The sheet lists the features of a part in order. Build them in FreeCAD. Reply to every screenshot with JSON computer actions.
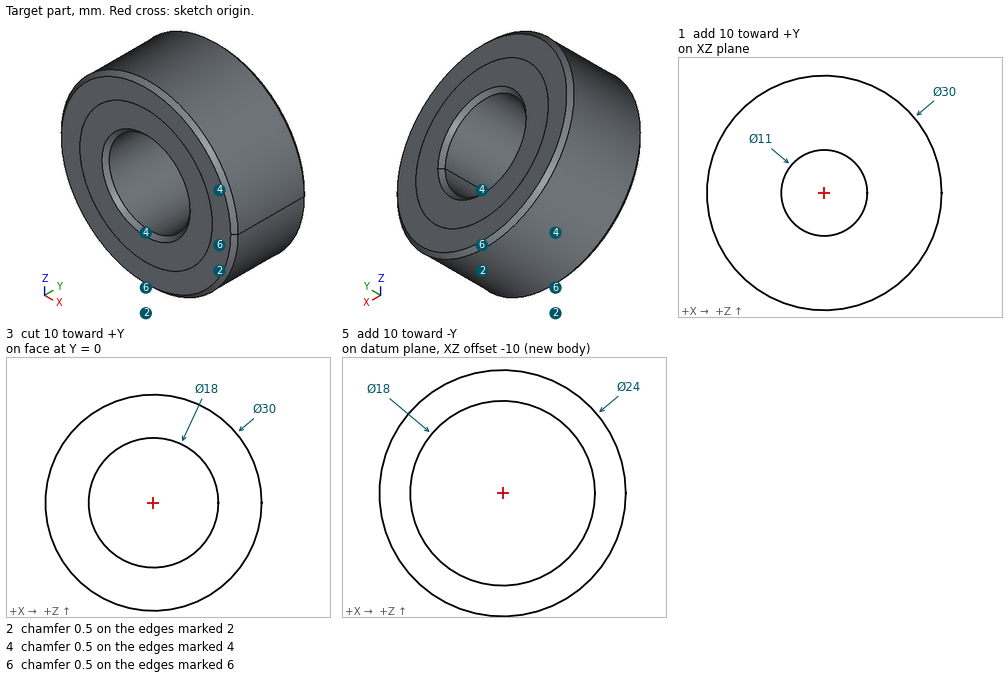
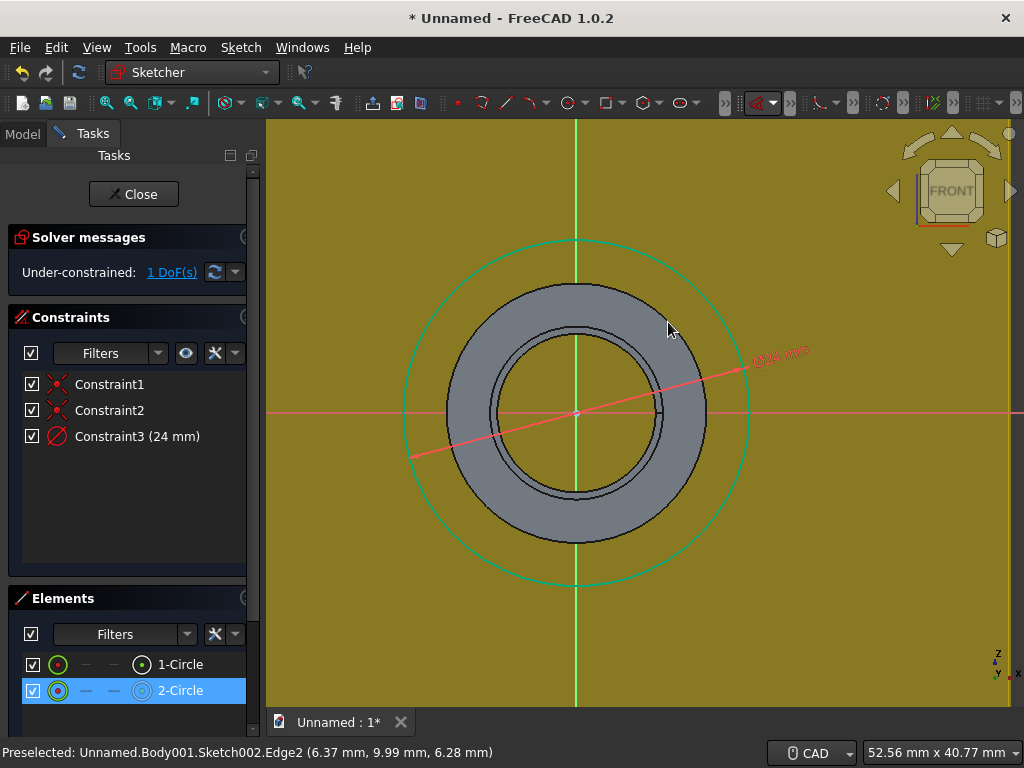
{"action": "left_click", "coordinate": [776, 104]}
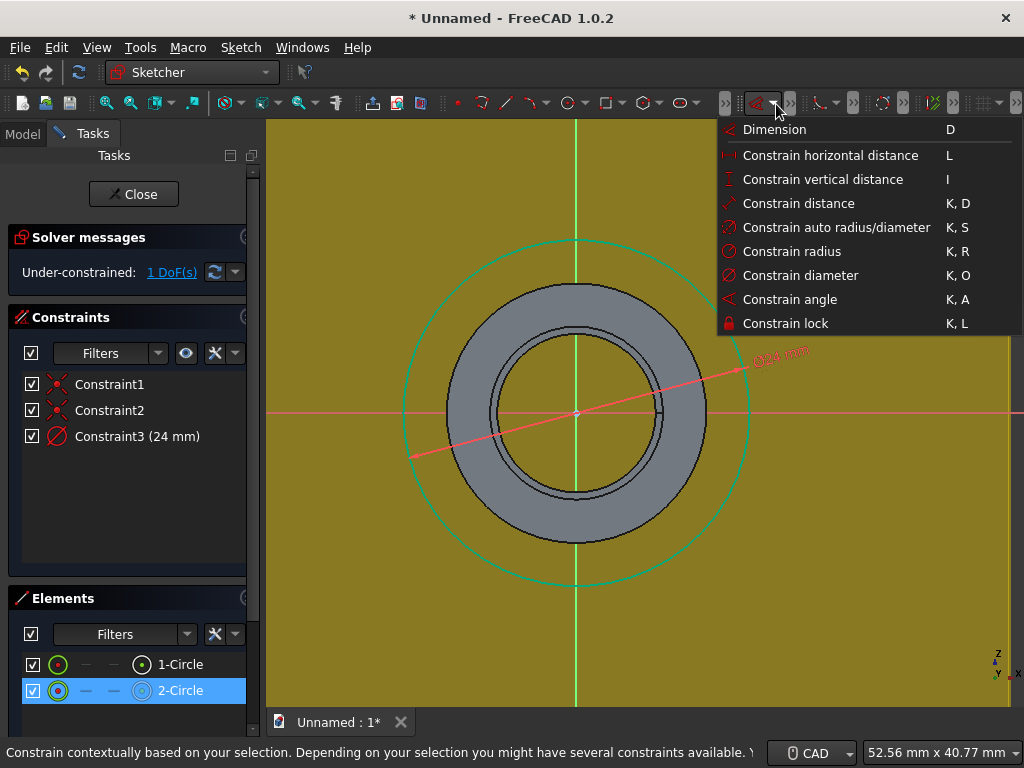
{"action": "left_click", "coordinate": [870, 275]}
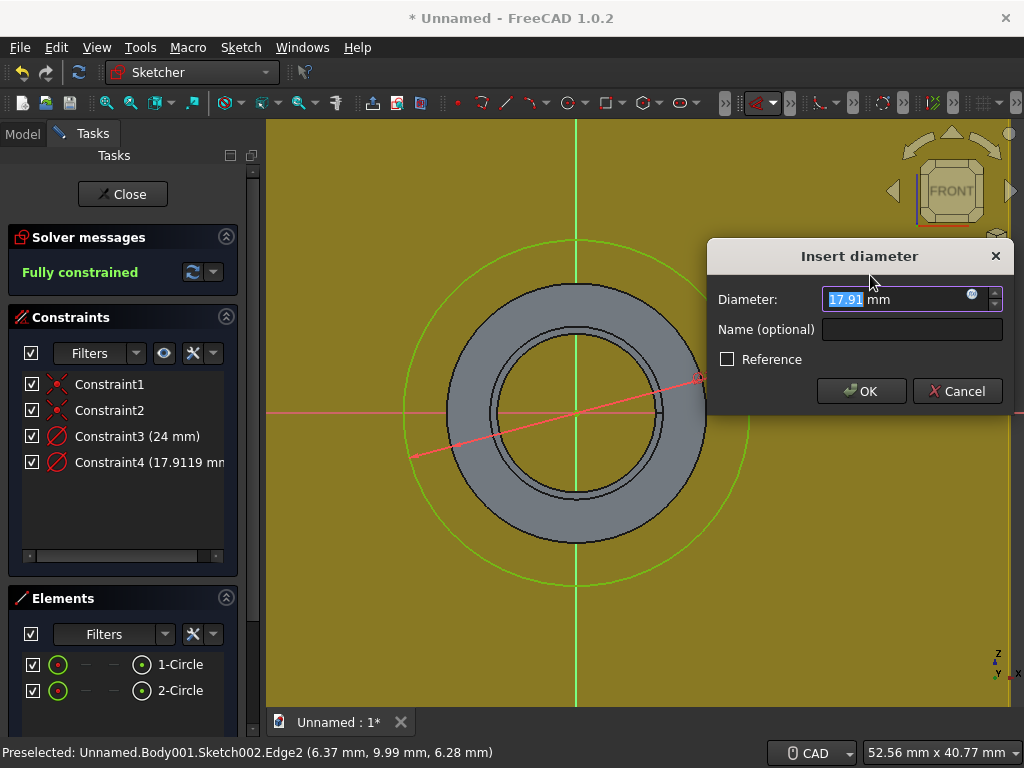
{"action": "type", "text": "18"}
{"action": "key", "text": "Return"}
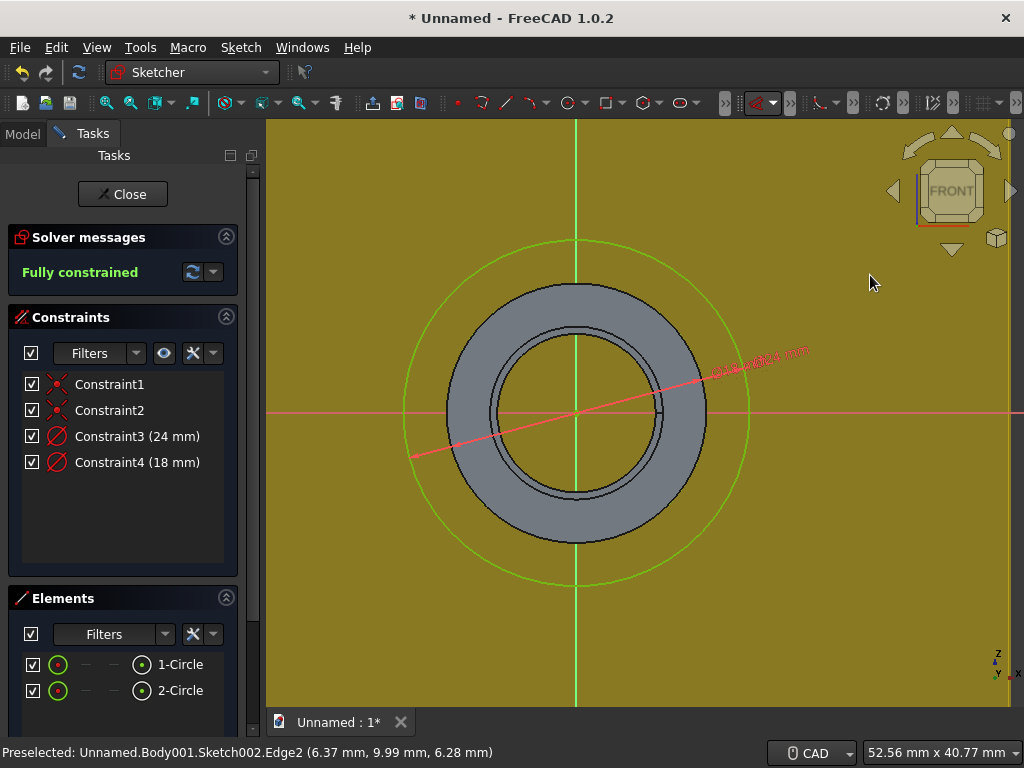
{"action": "left_click", "coordinate": [123, 194]}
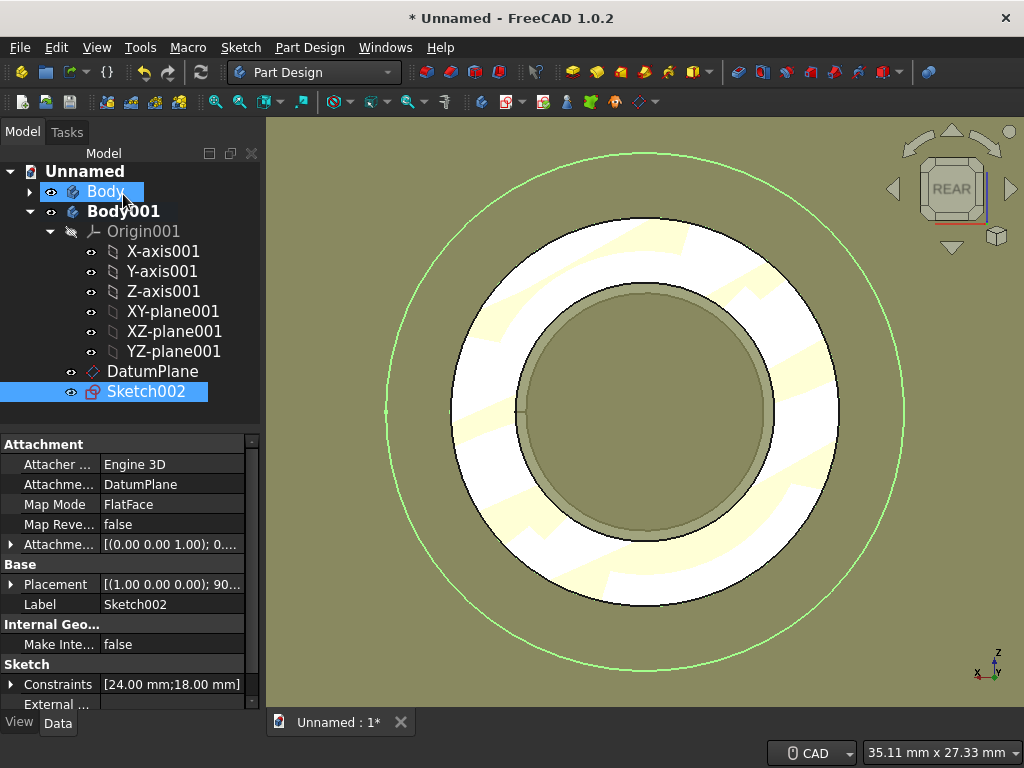
{"action": "left_click", "coordinate": [574, 72]}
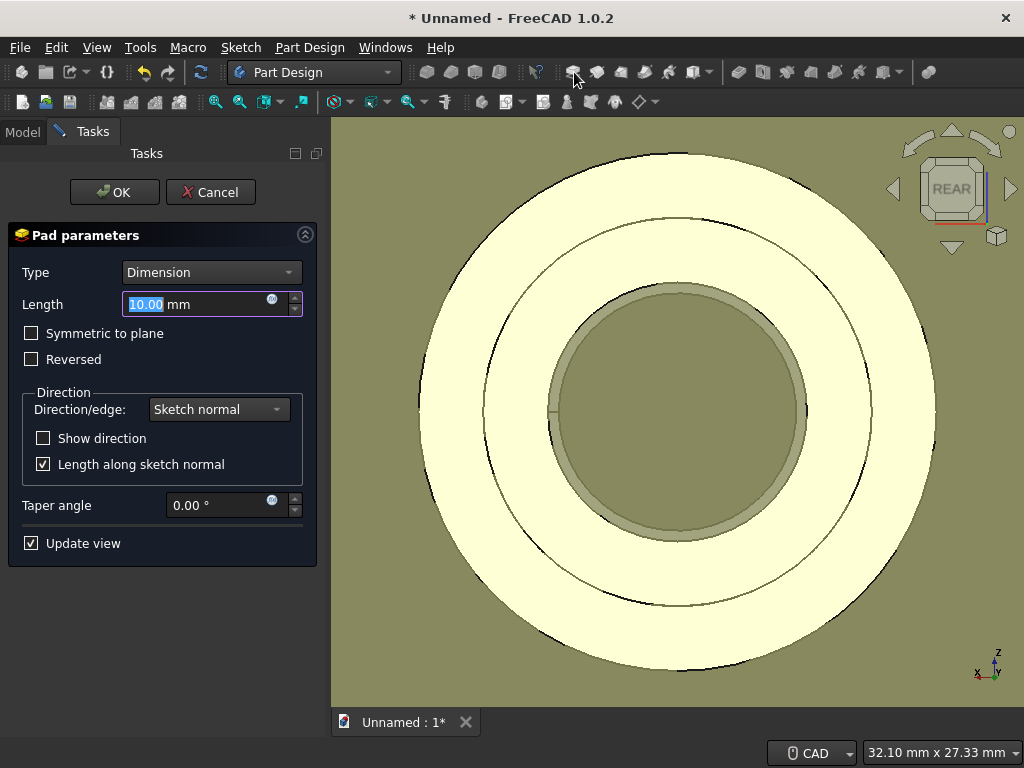
{"action": "type", "text": "10"}
{"action": "key", "text": "Tab"}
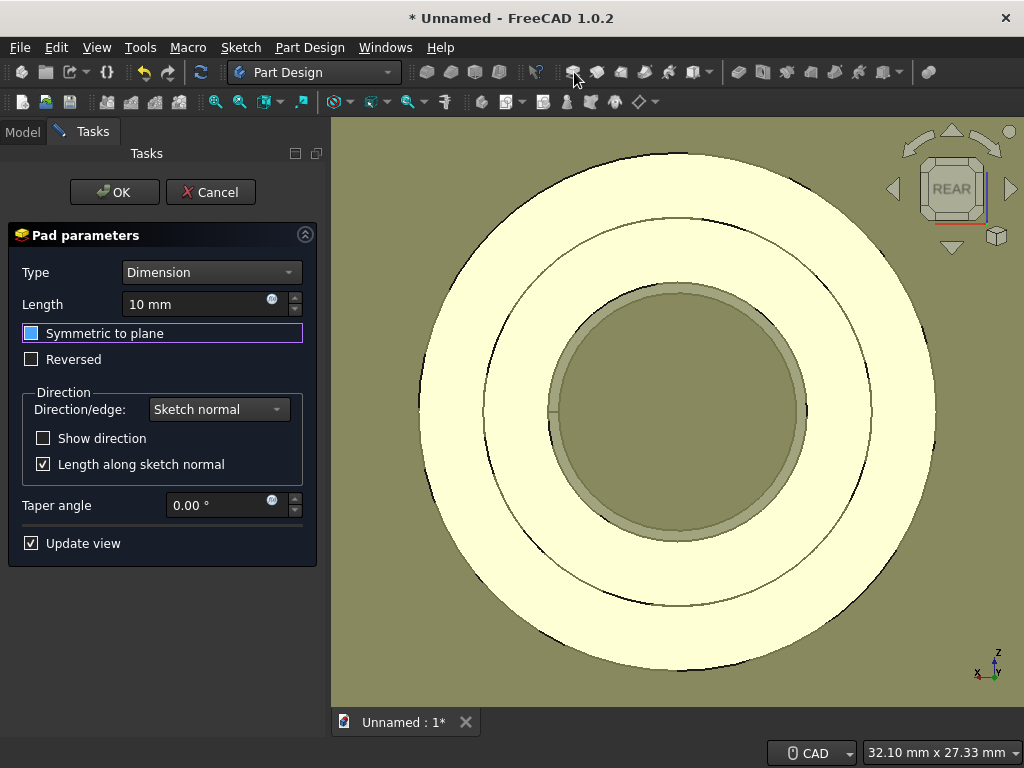
{"action": "left_click", "coordinate": [115, 192]}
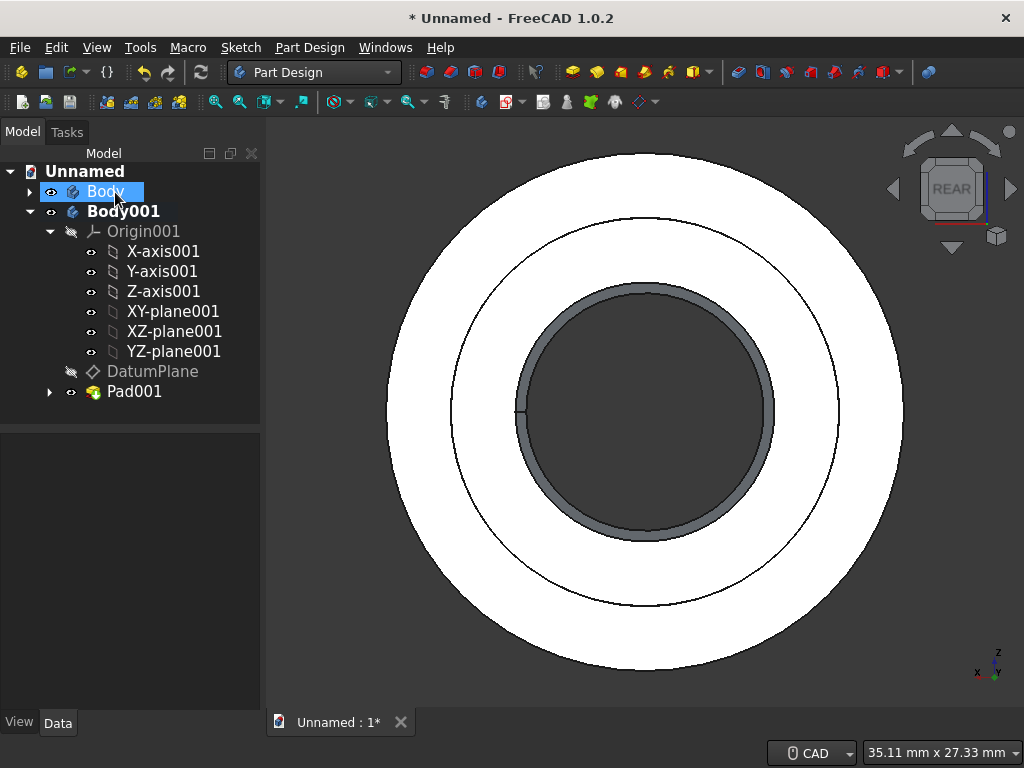
{"action": "left_click", "coordinate": [904, 411]}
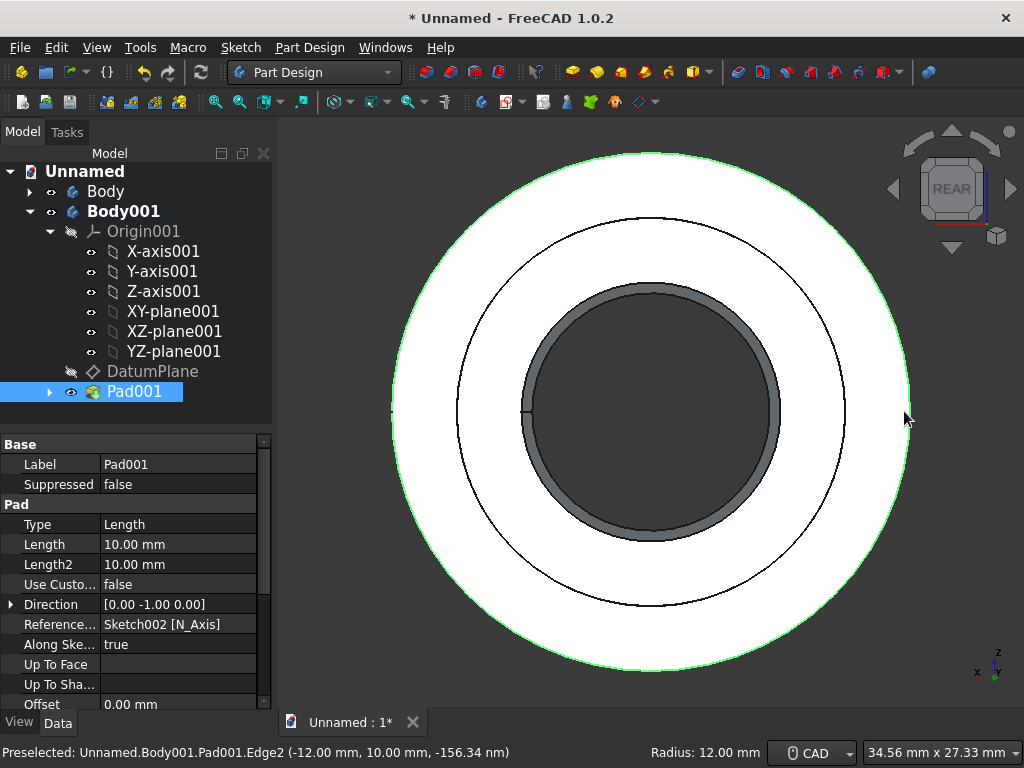
{"action": "key", "text": "0"}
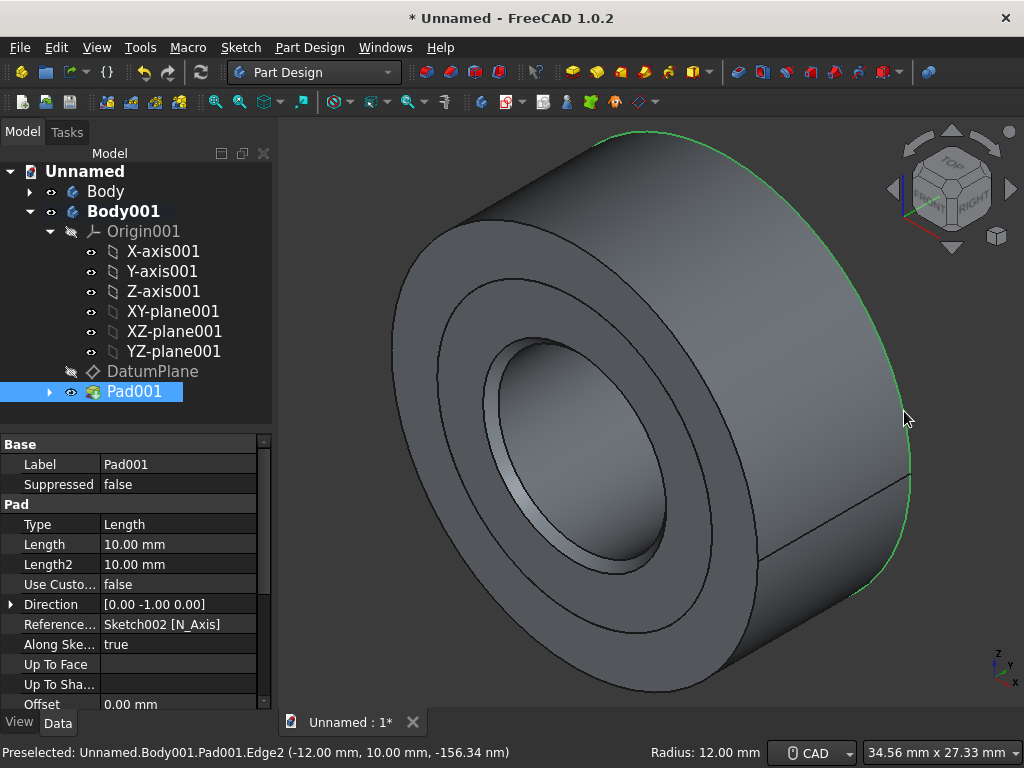
{"action": "left_click", "coordinate": [216, 102]}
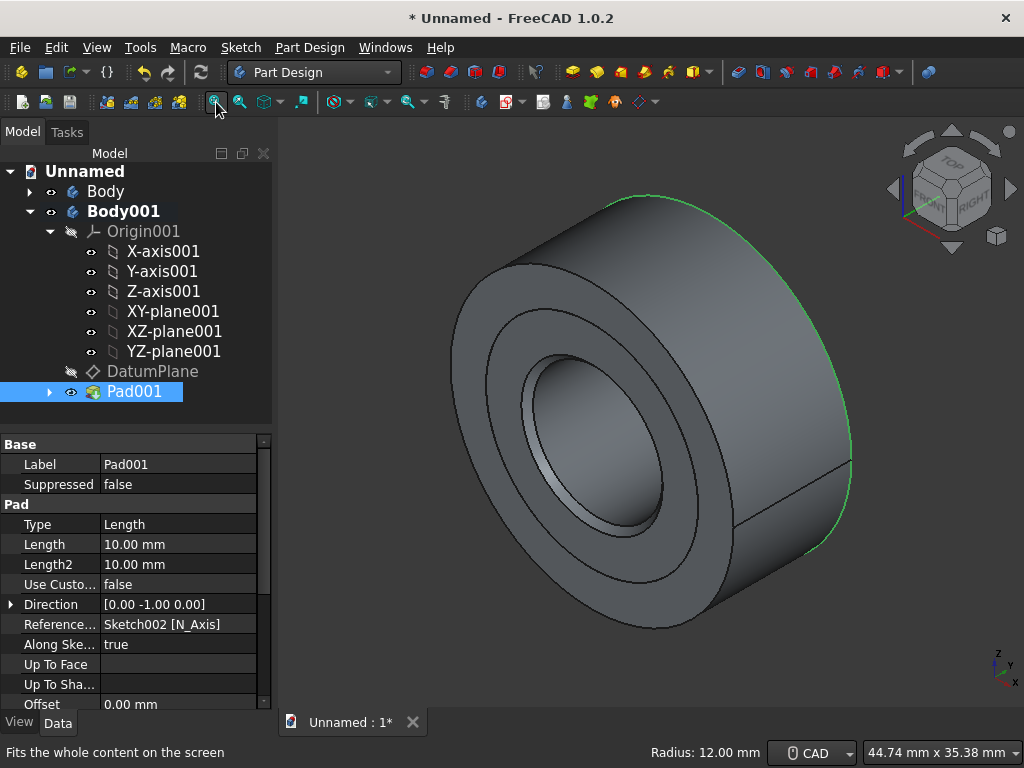
{"action": "left_click", "coordinate": [548, 264], "text": "ctrl"}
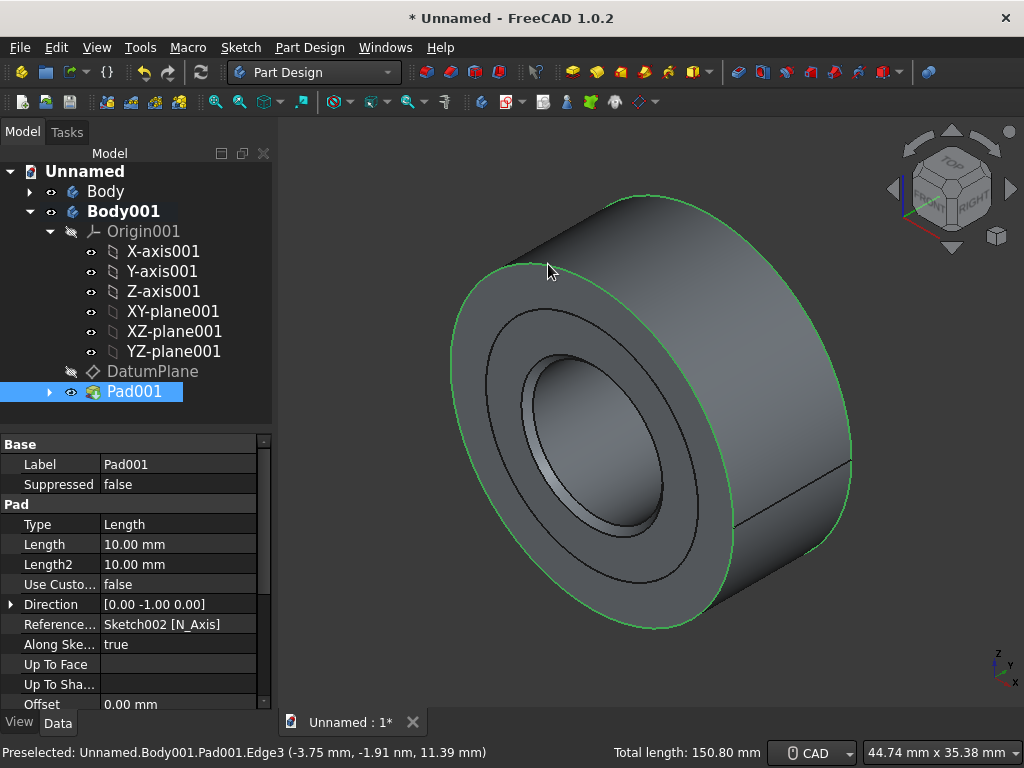
{"action": "left_click", "coordinate": [452, 72]}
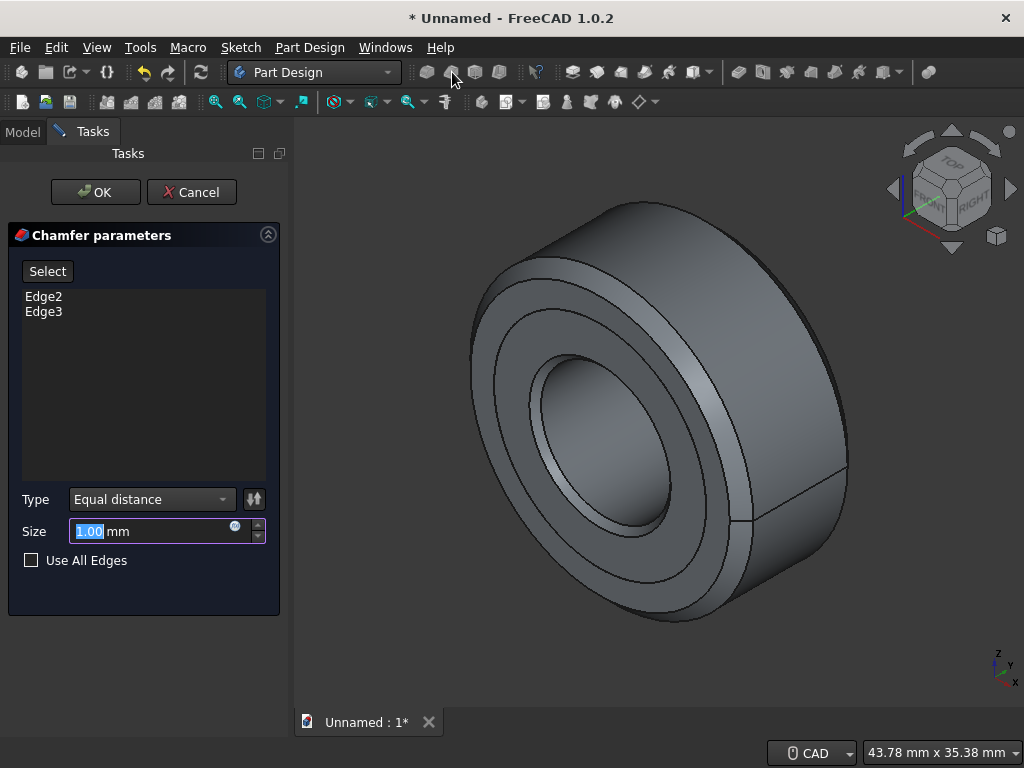
{"action": "type", "text": "0.5"}
{"action": "key", "text": "Tab"}